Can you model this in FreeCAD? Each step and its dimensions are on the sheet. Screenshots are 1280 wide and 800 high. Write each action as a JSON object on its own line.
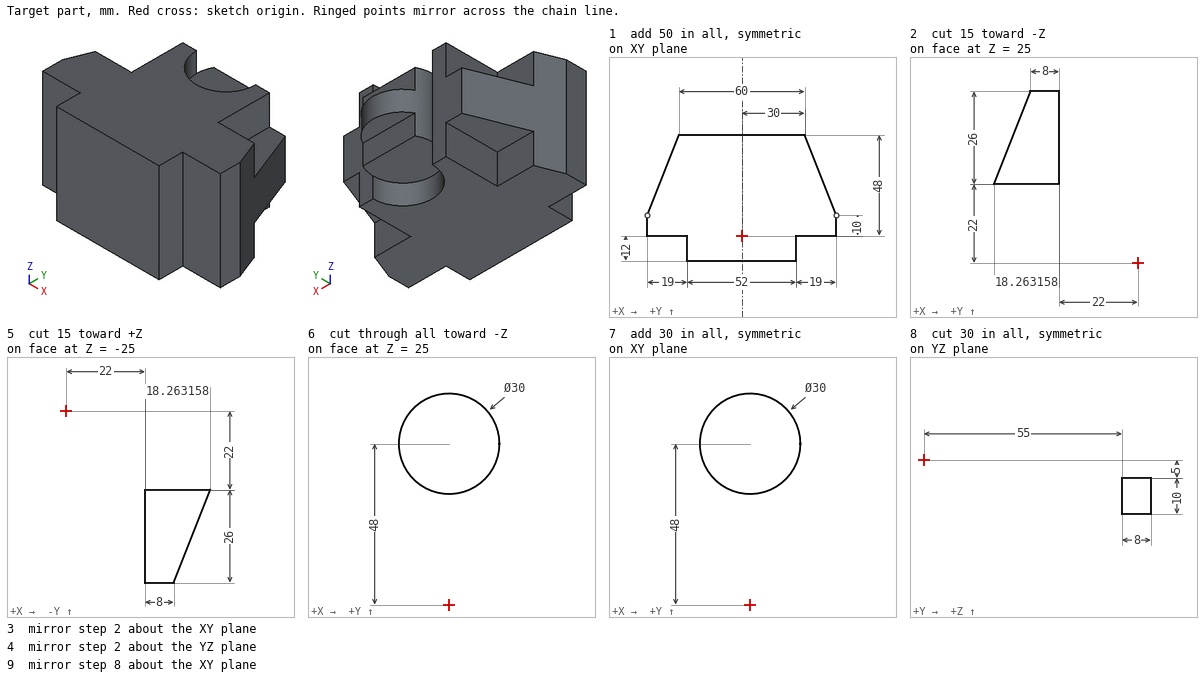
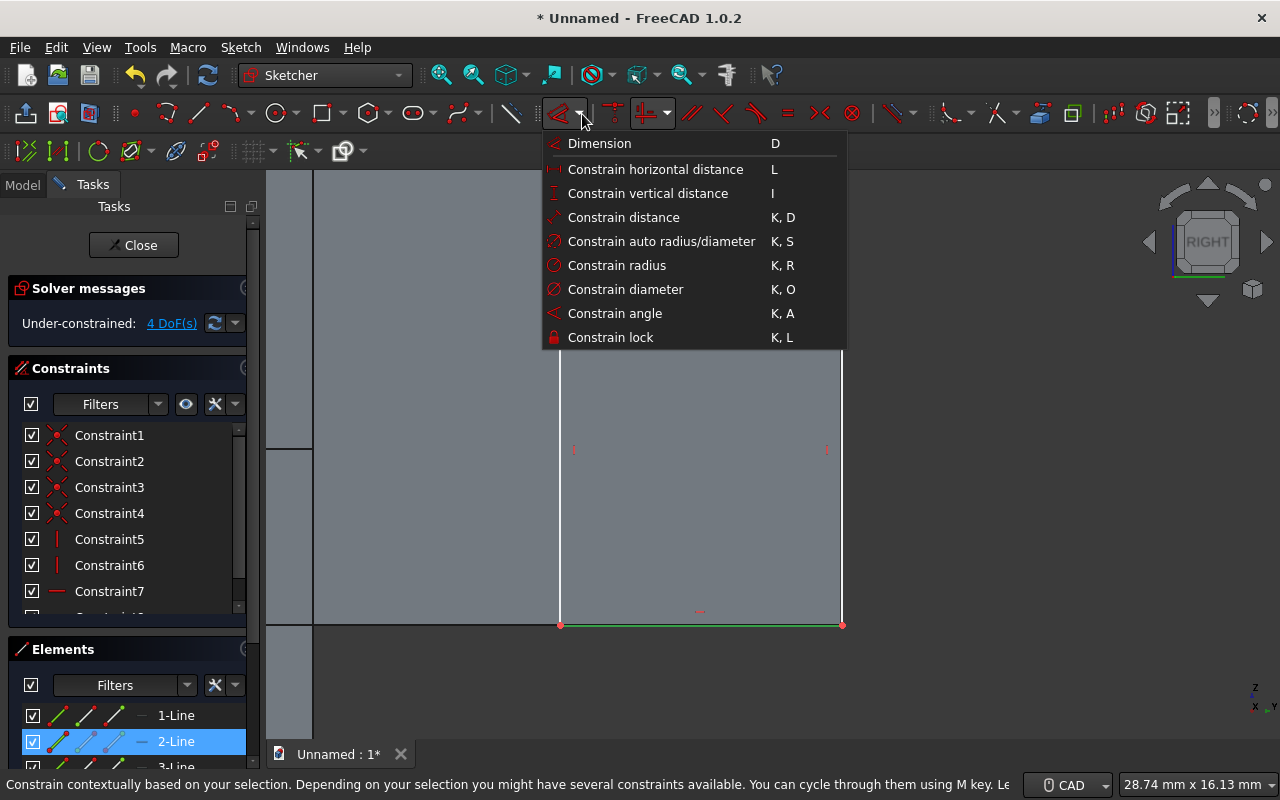
{"action": "left_click", "coordinate": [695, 169]}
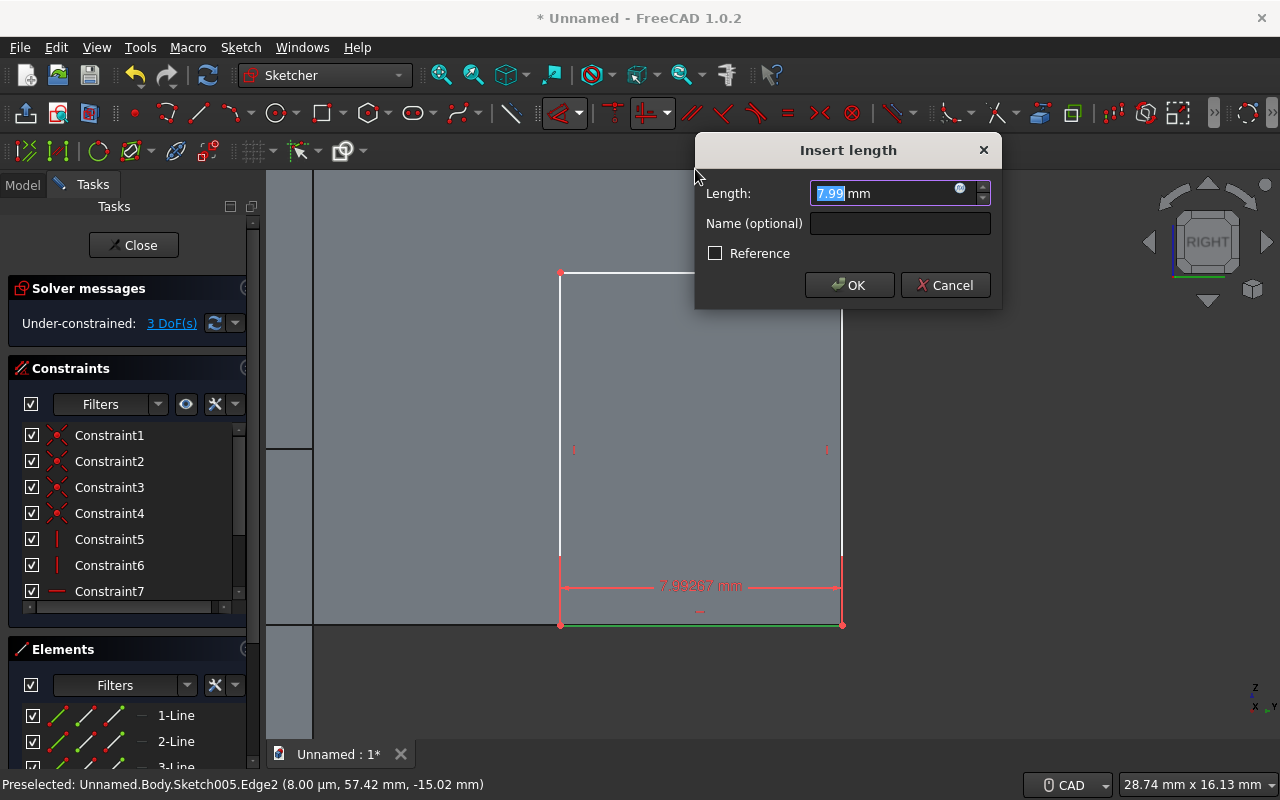
{"action": "type", "text": "8"}
{"action": "key", "text": "Return"}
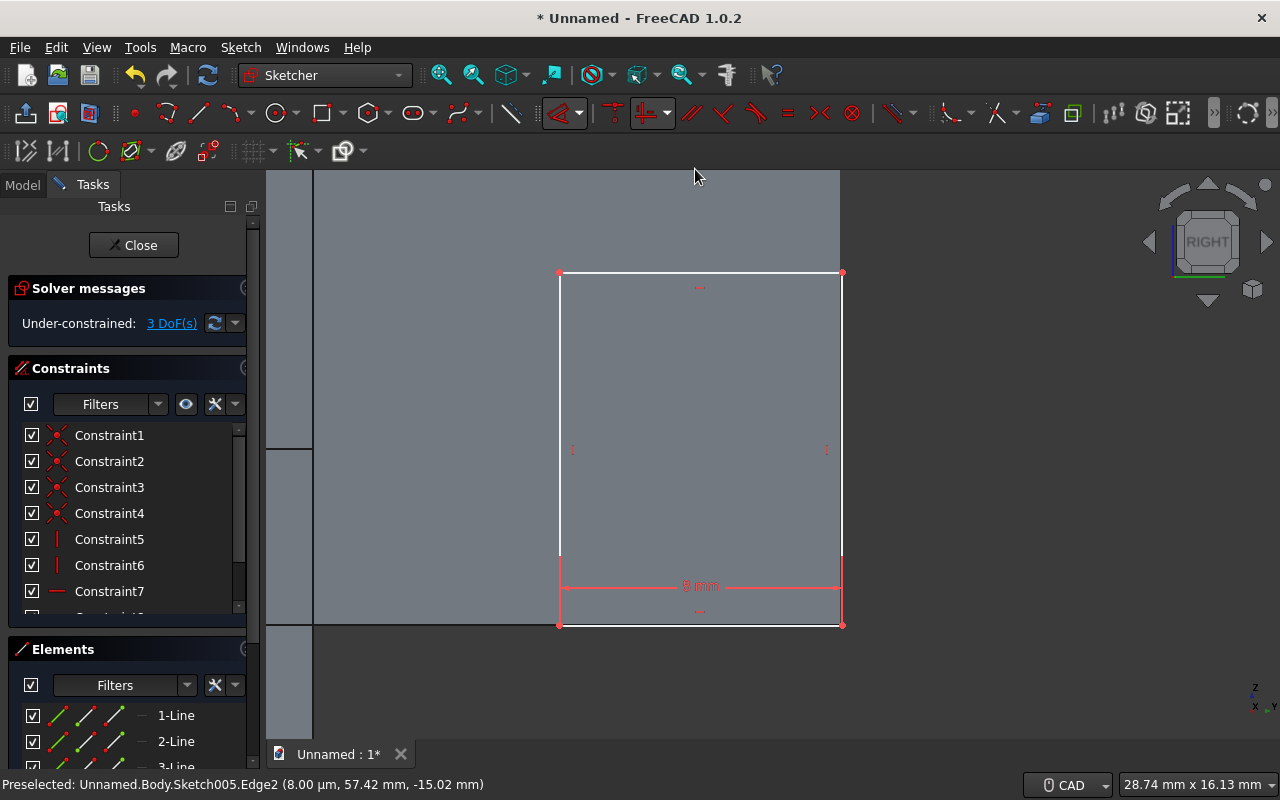
{"action": "left_click", "coordinate": [560, 379]}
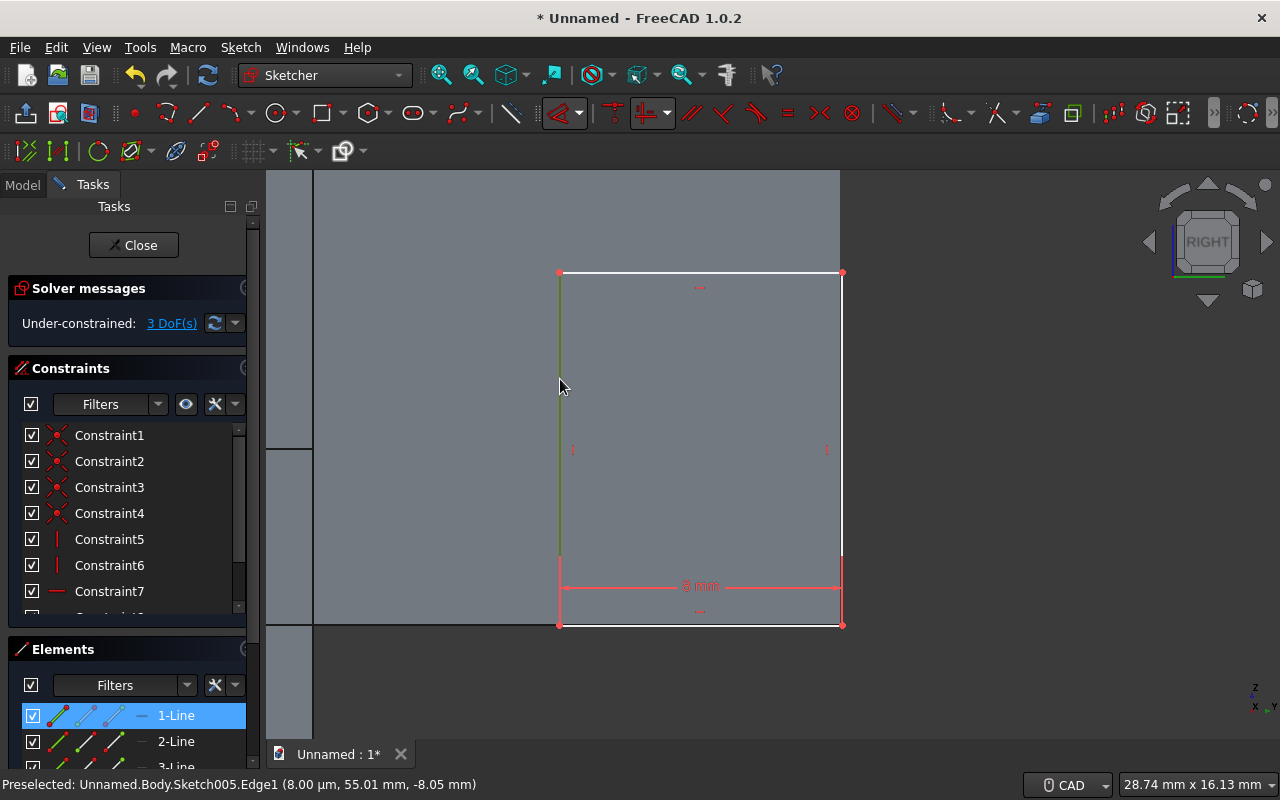
{"action": "key", "text": "i"}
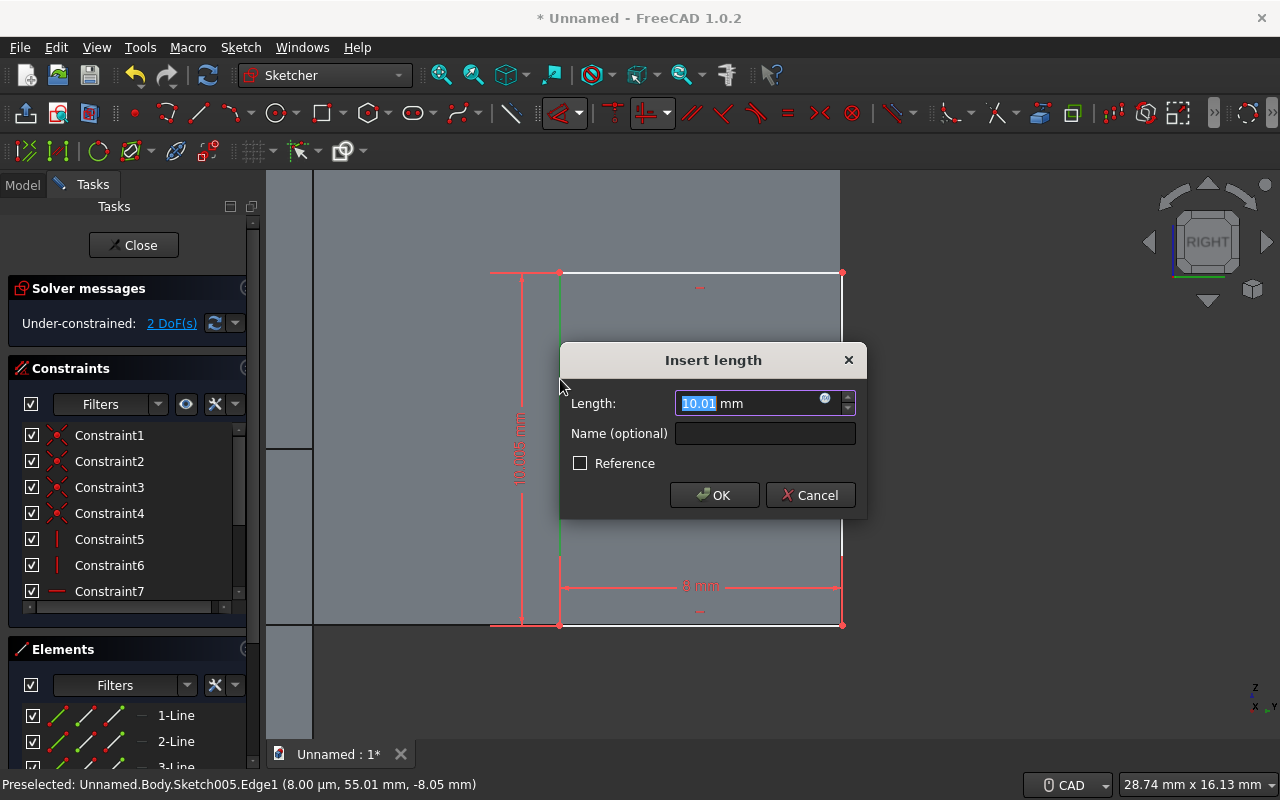
{"action": "type", "text": "10"}
{"action": "key", "text": "Return"}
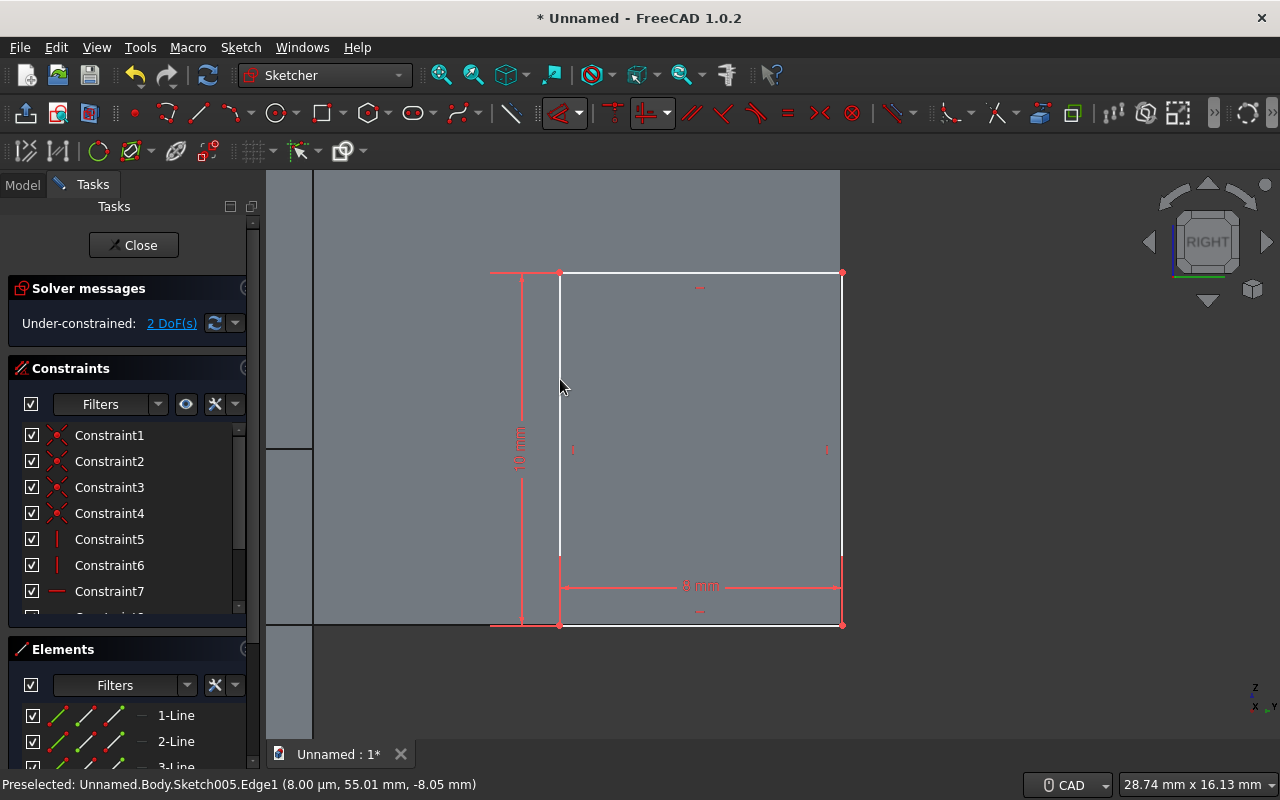
{"action": "left_click", "coordinate": [560, 273]}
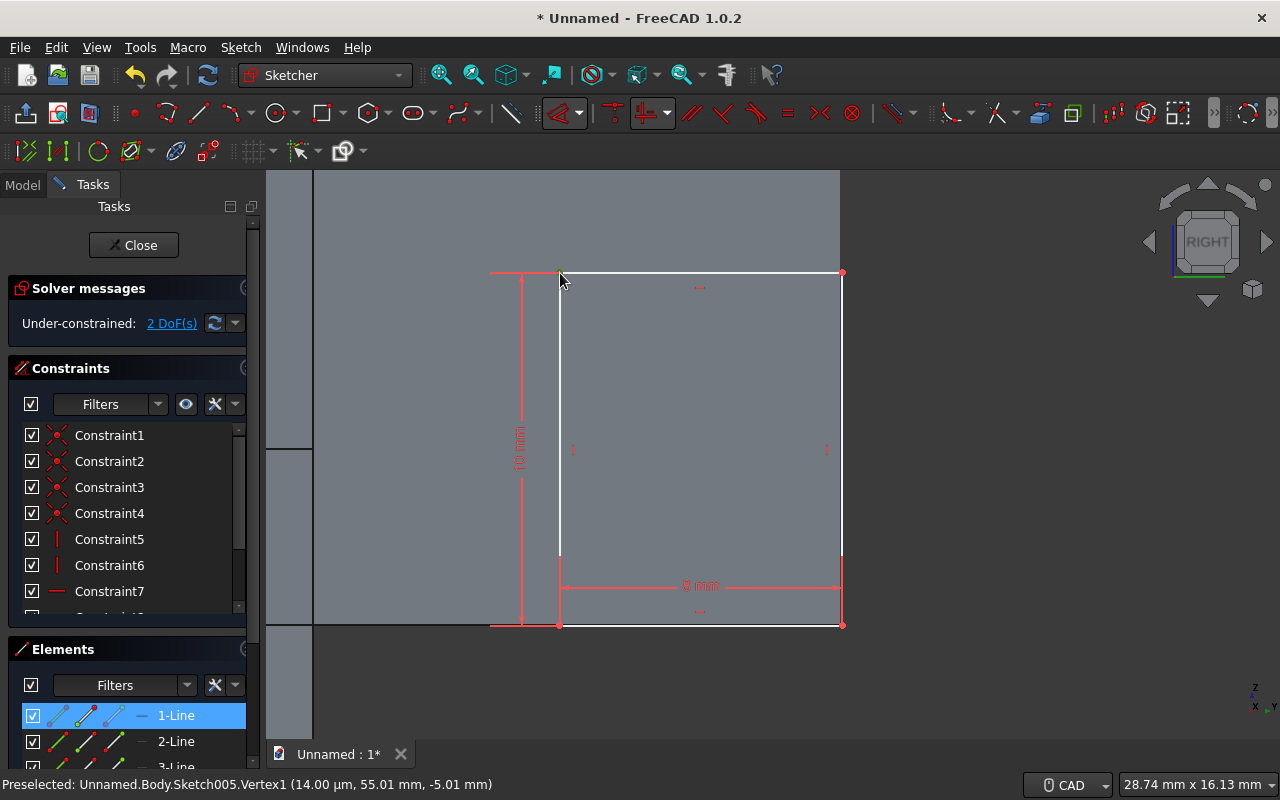
{"action": "key", "text": "i"}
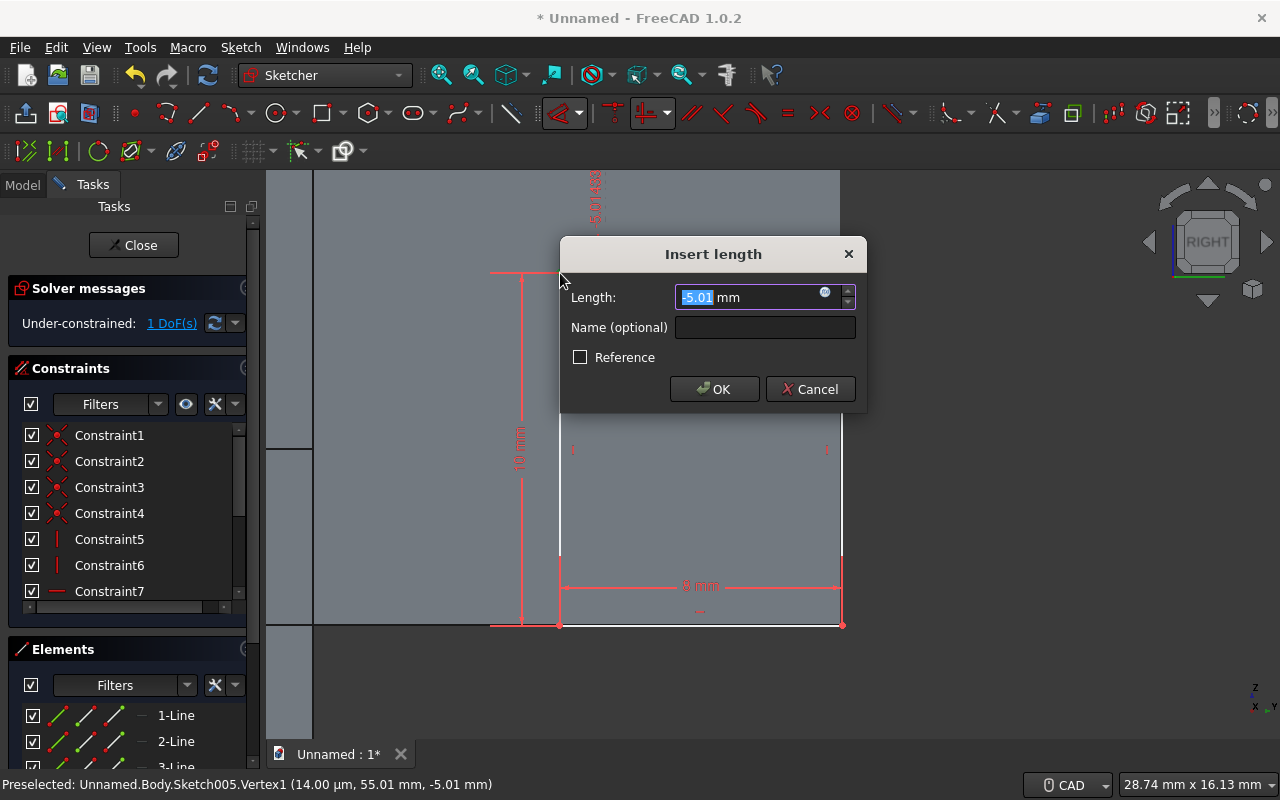
{"action": "type", "text": "-5"}
{"action": "key", "text": "Return"}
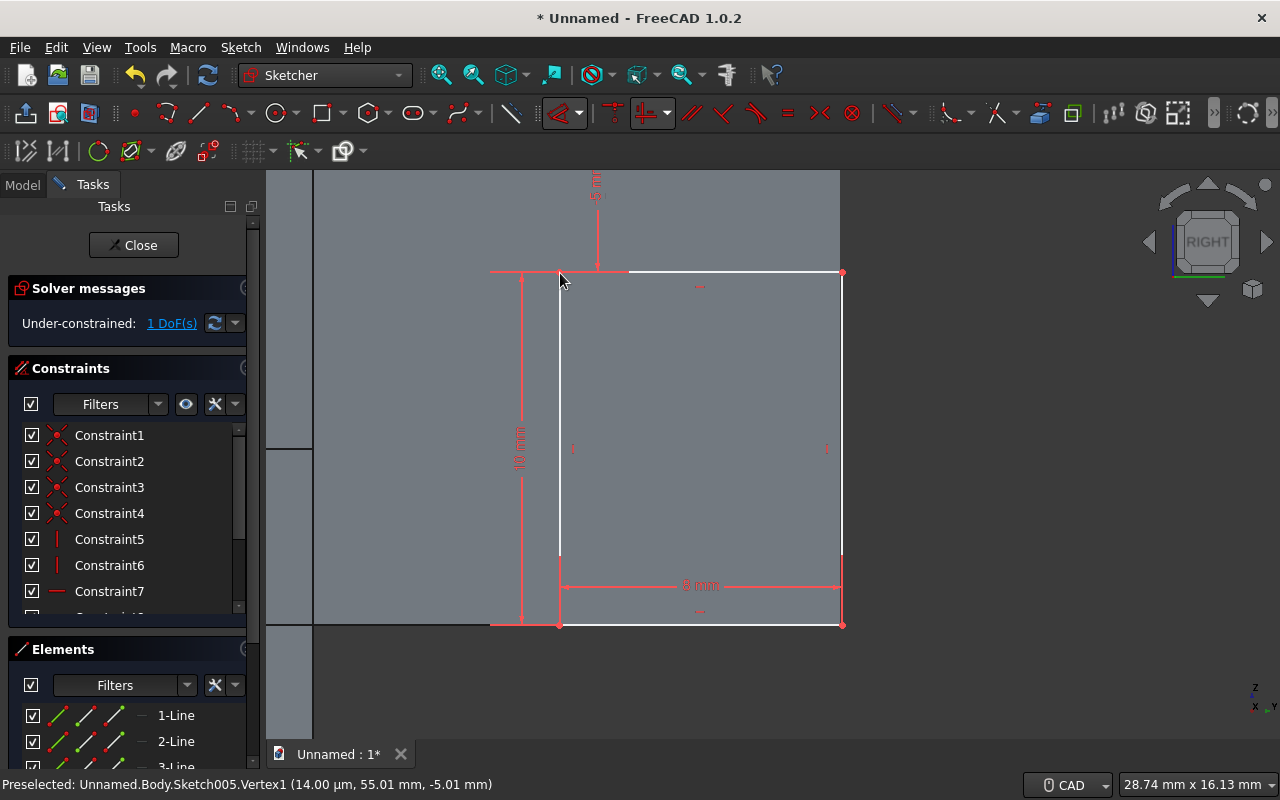
{"action": "left_click", "coordinate": [560, 272]}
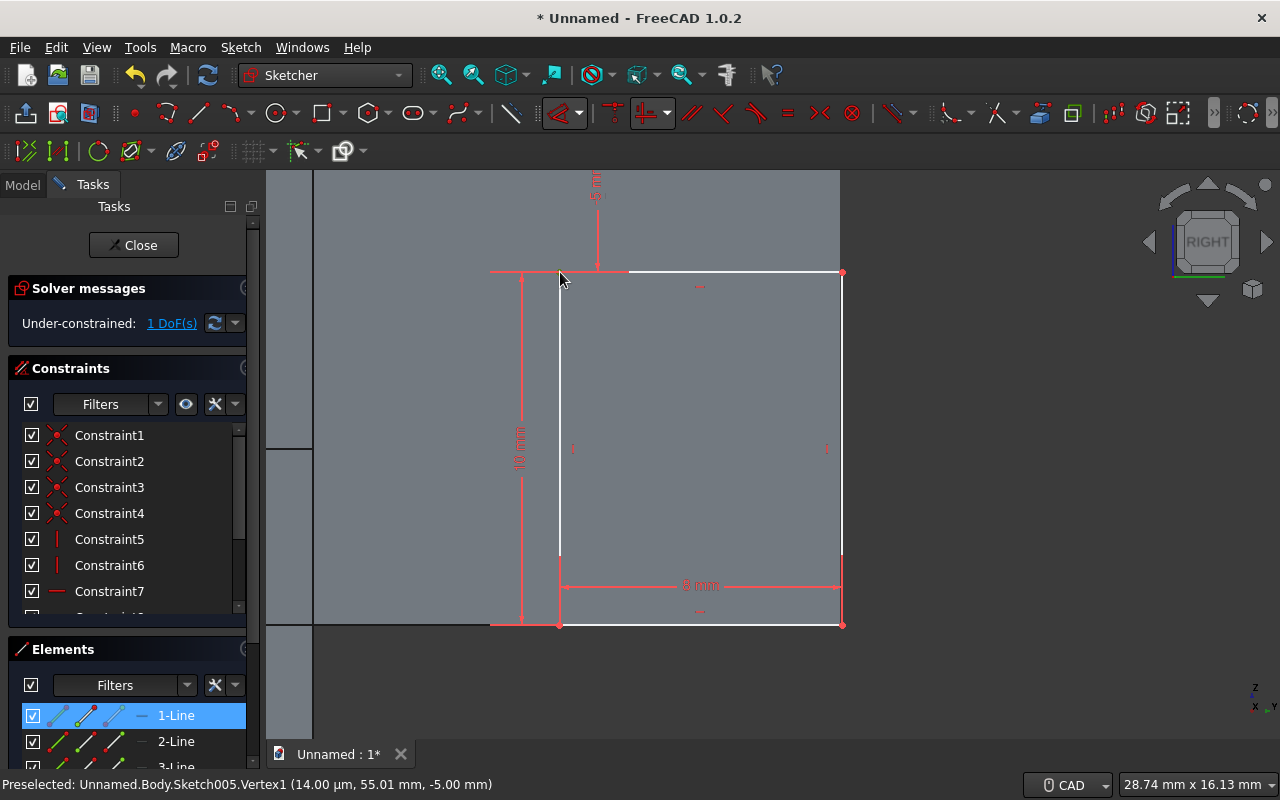
{"action": "left_click", "coordinate": [582, 114]}